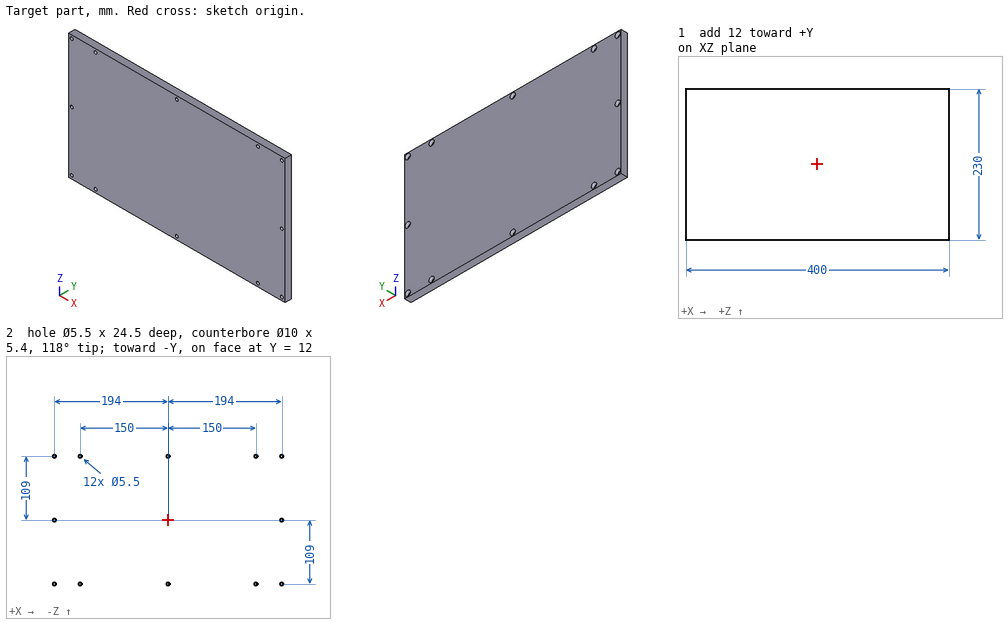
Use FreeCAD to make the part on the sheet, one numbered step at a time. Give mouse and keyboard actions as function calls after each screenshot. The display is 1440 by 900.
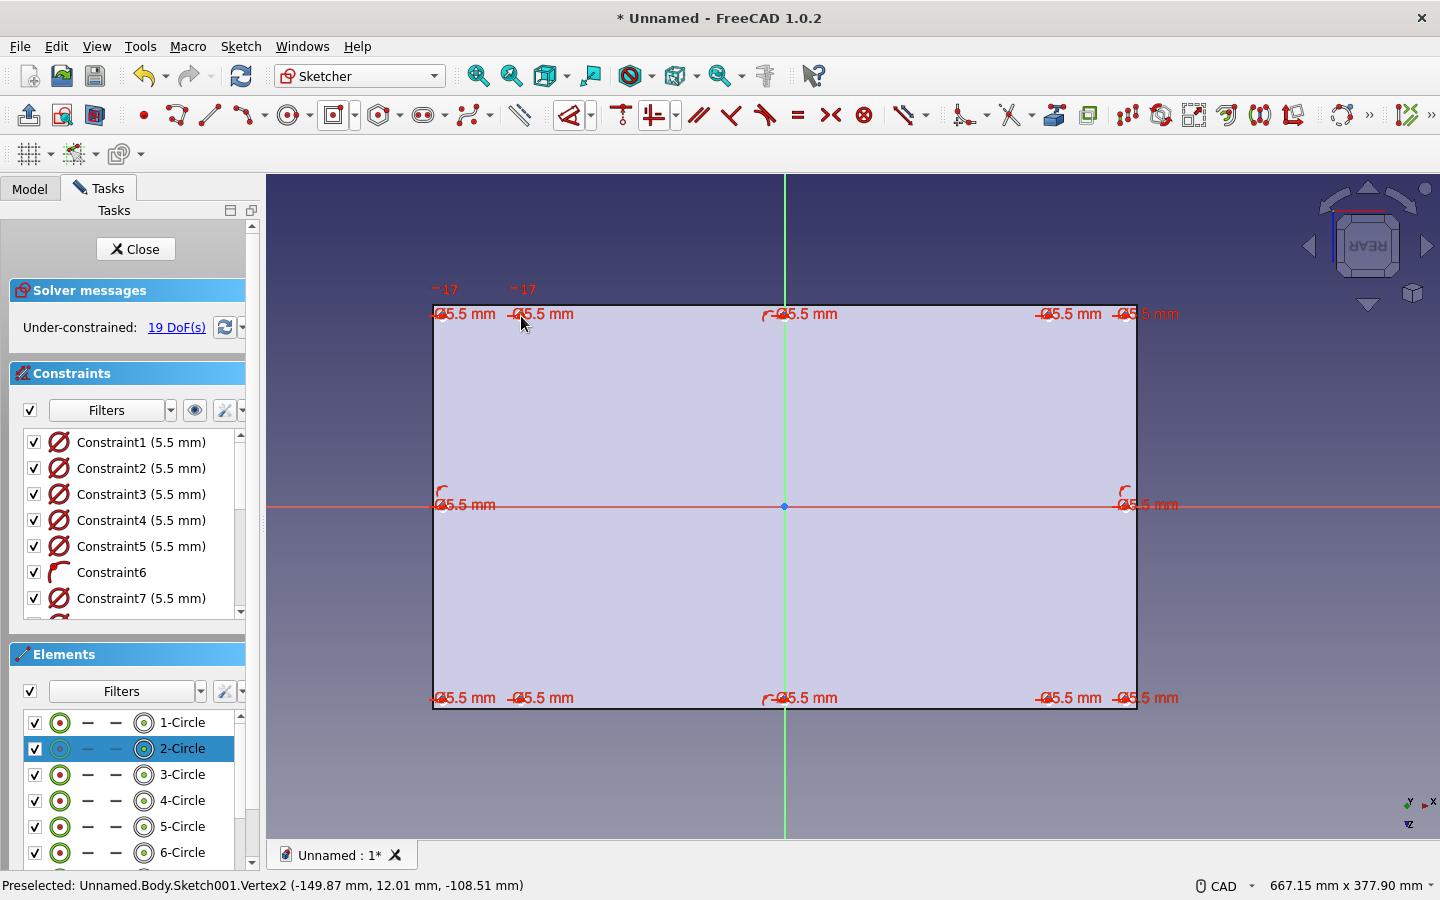
click(1049, 316)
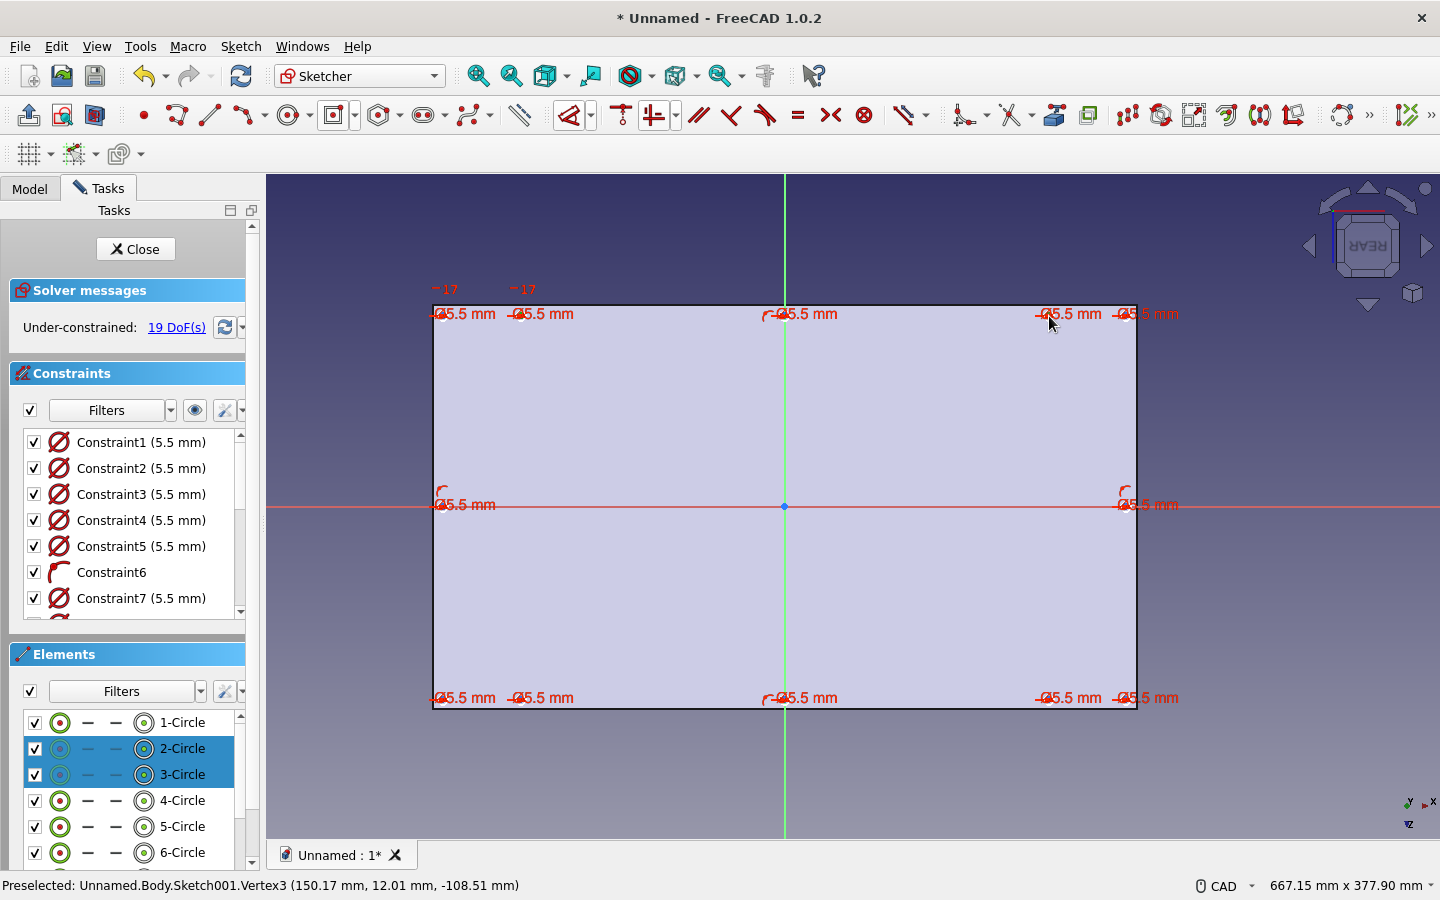
click(676, 116)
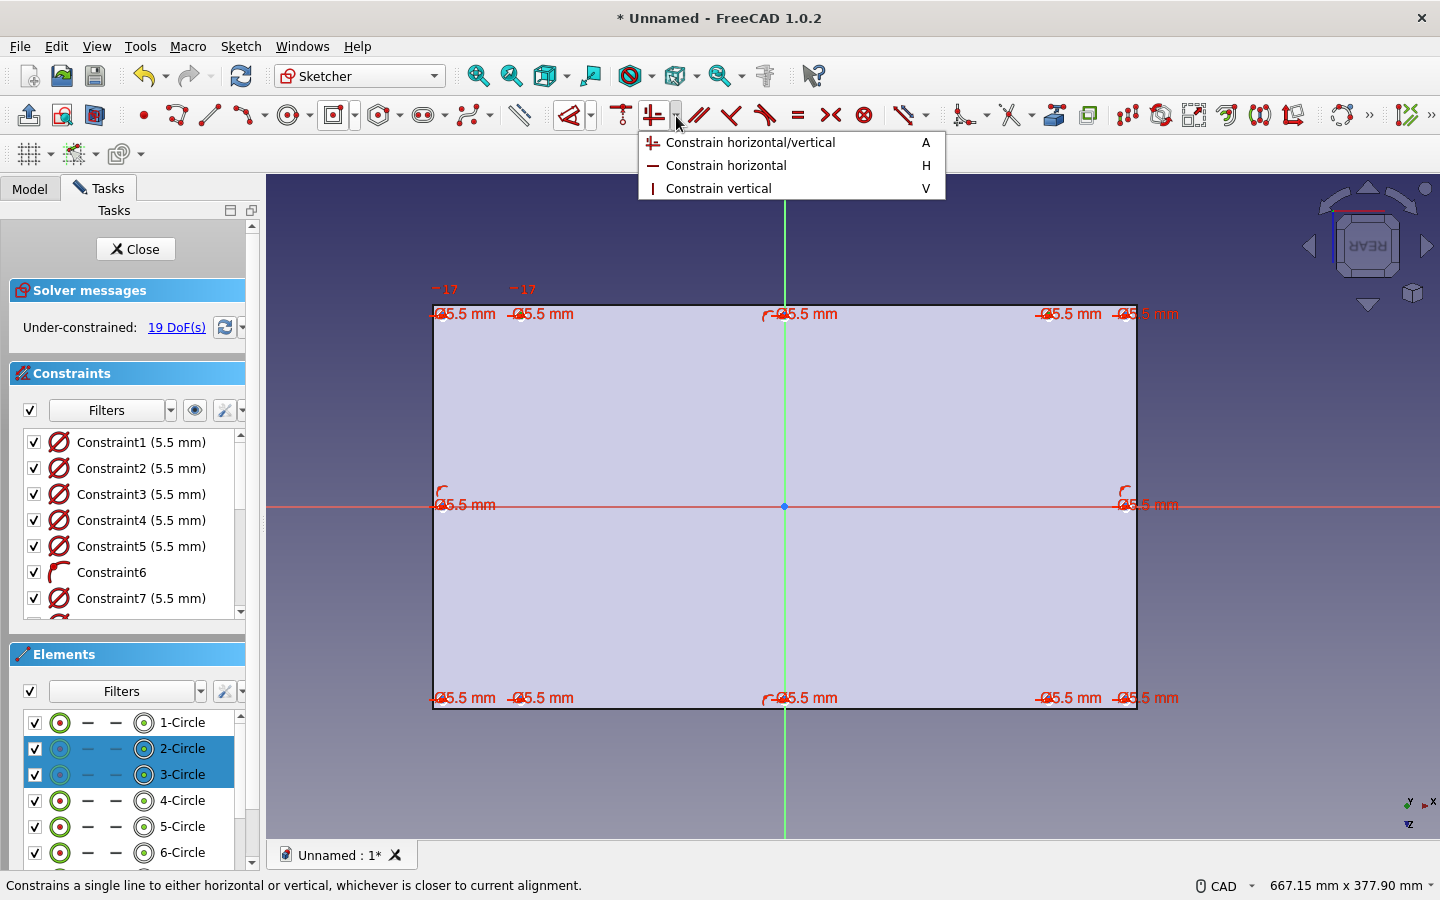
click(792, 166)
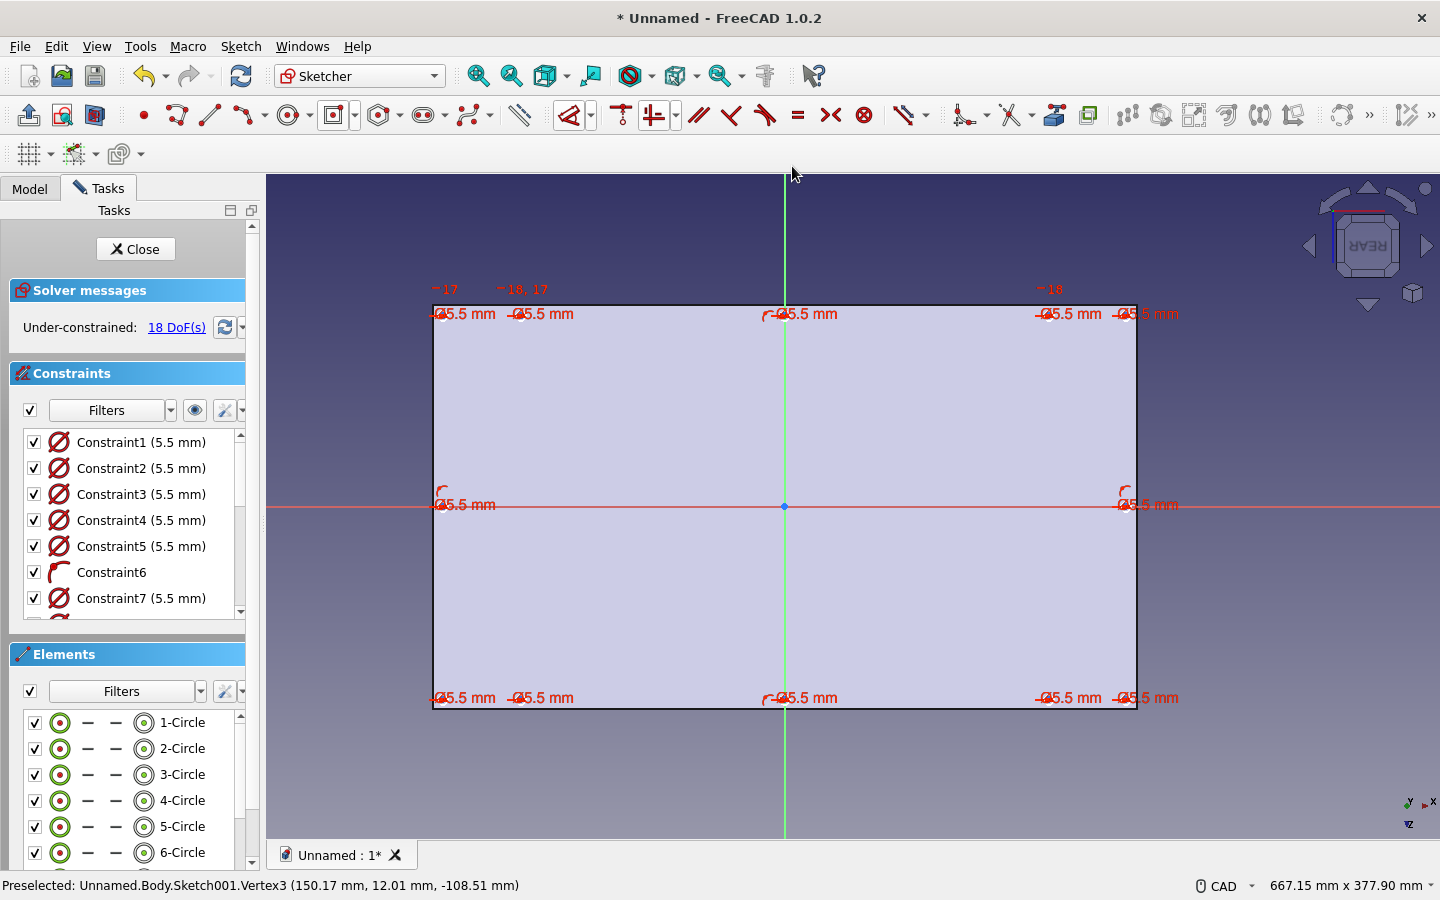
click(1049, 316)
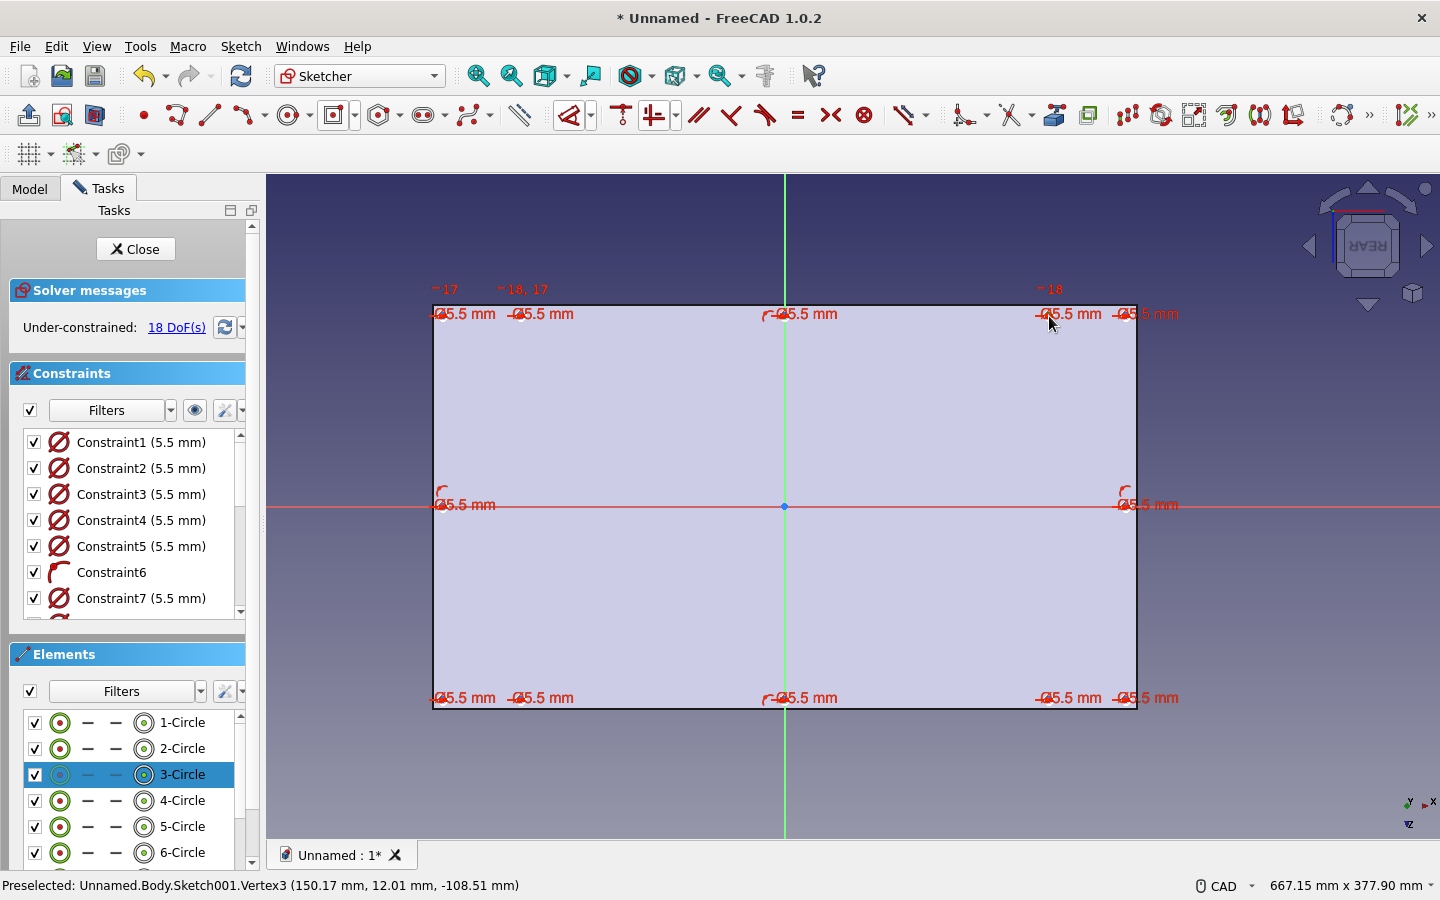
click(1126, 316)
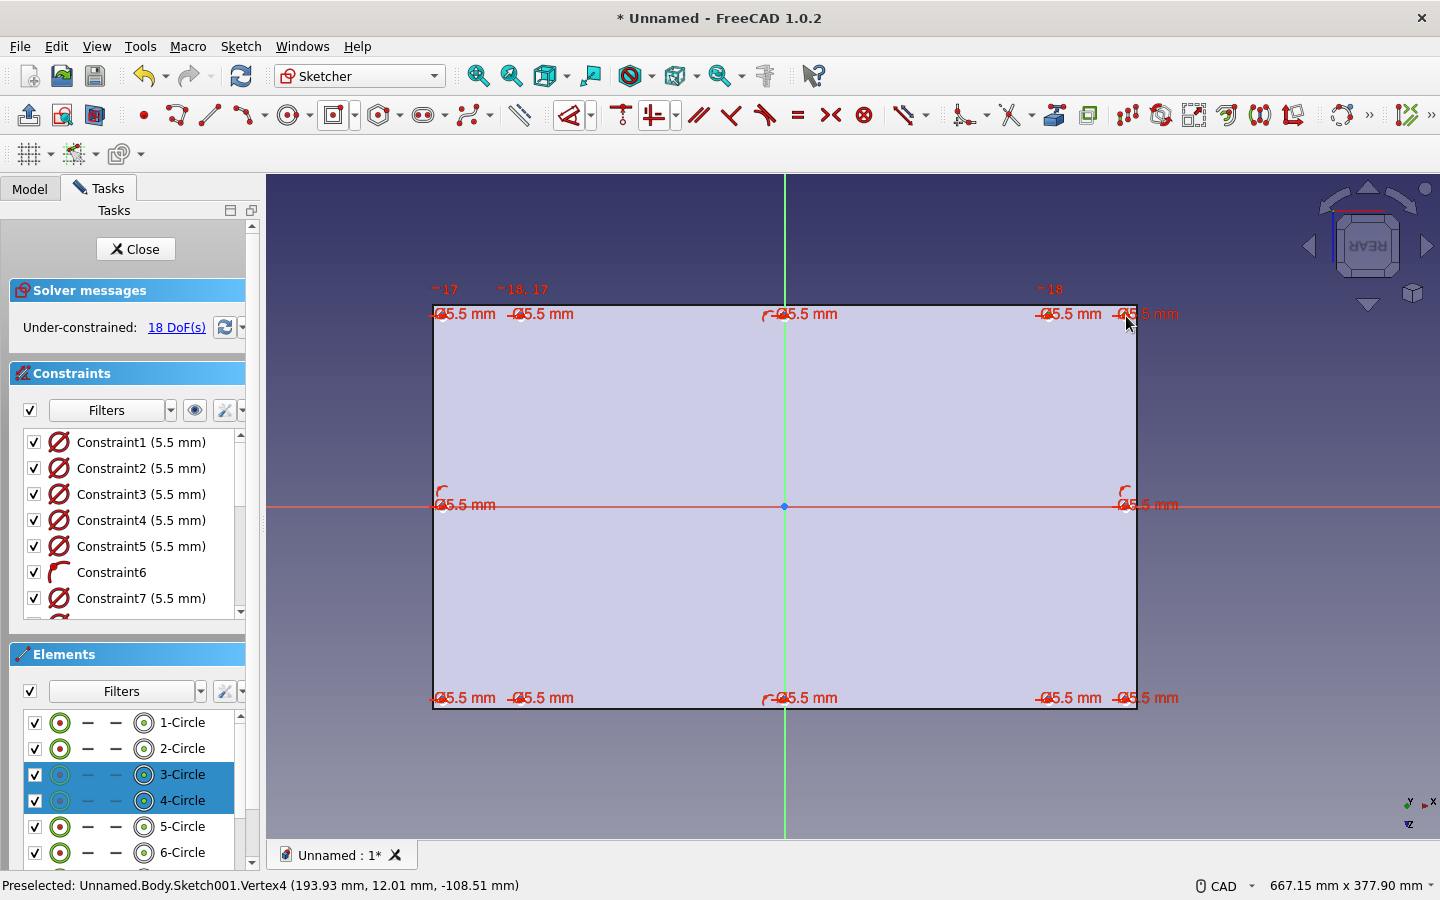
click(676, 116)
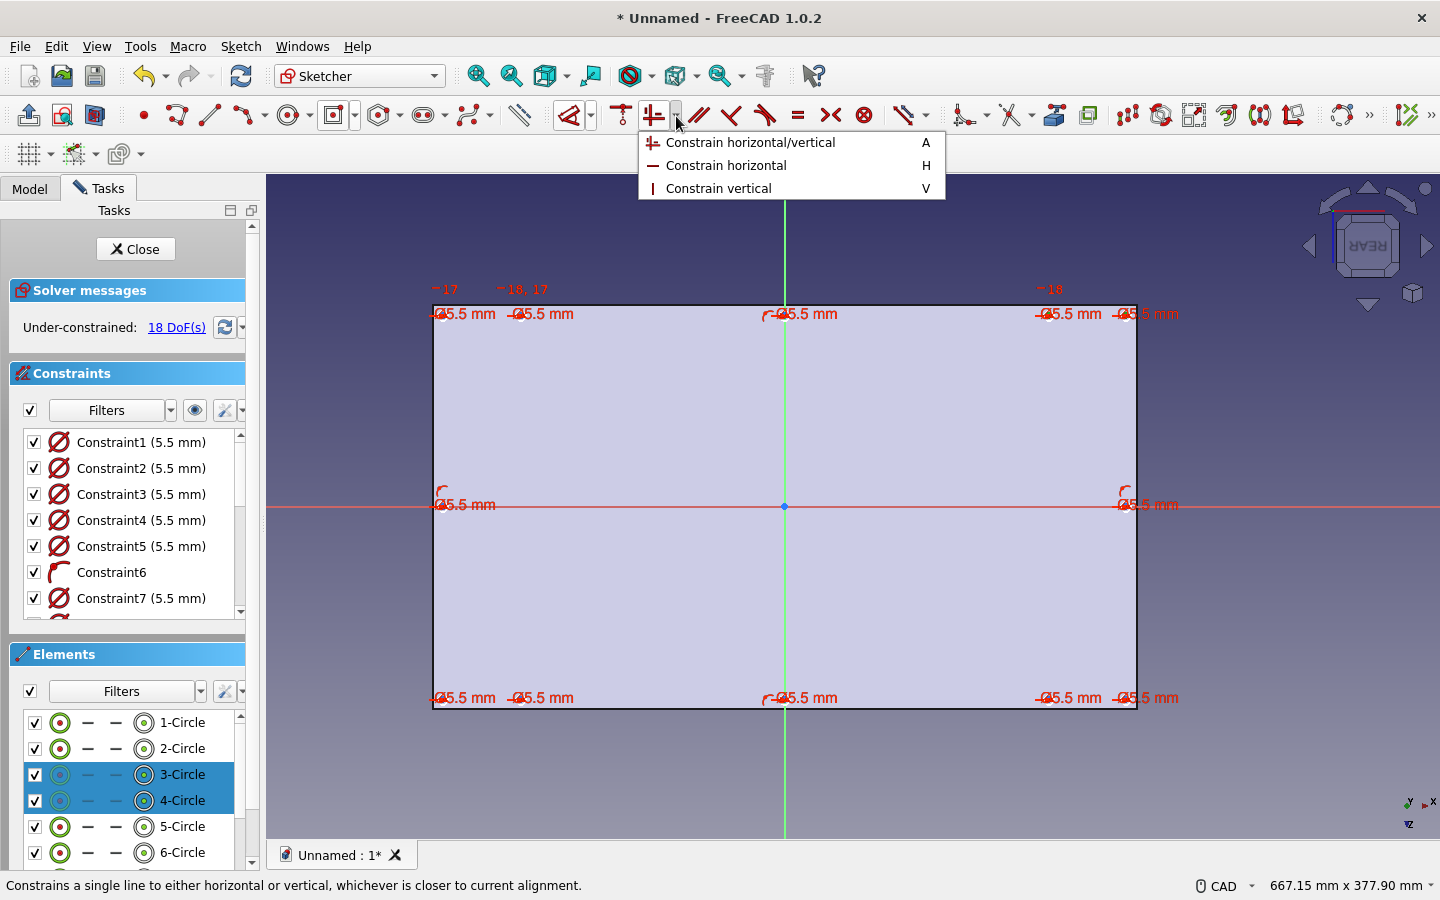
click(792, 166)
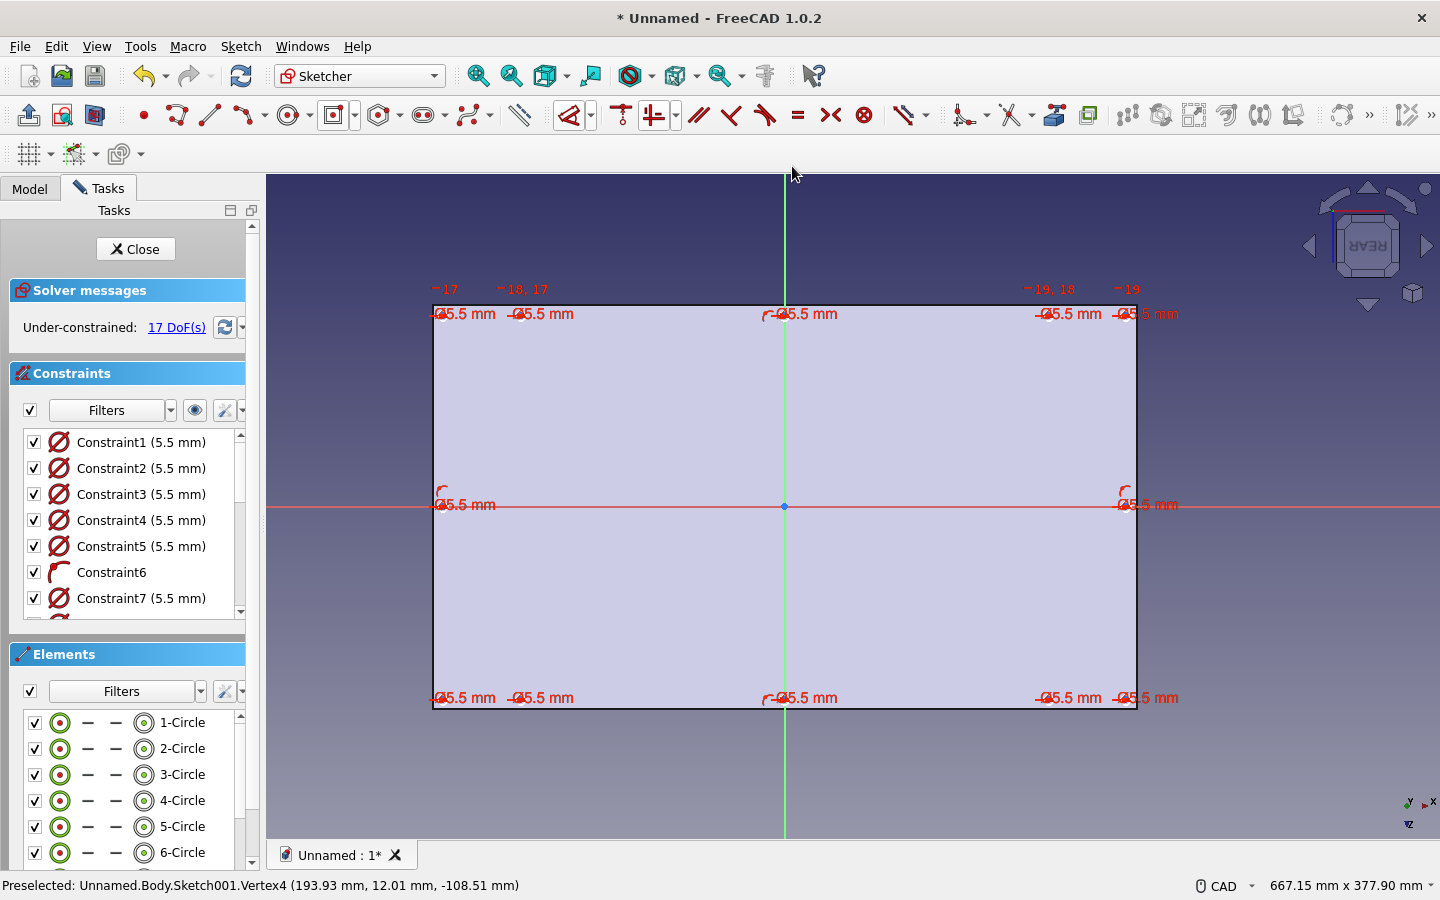
click(1126, 316)